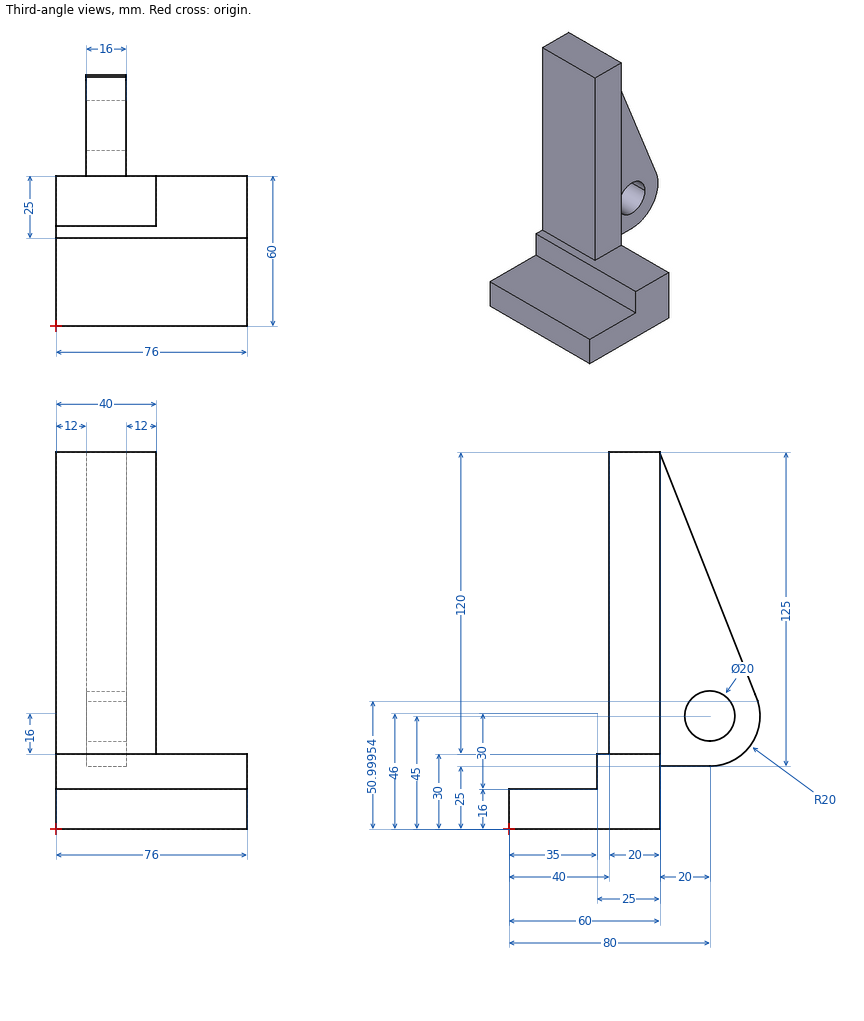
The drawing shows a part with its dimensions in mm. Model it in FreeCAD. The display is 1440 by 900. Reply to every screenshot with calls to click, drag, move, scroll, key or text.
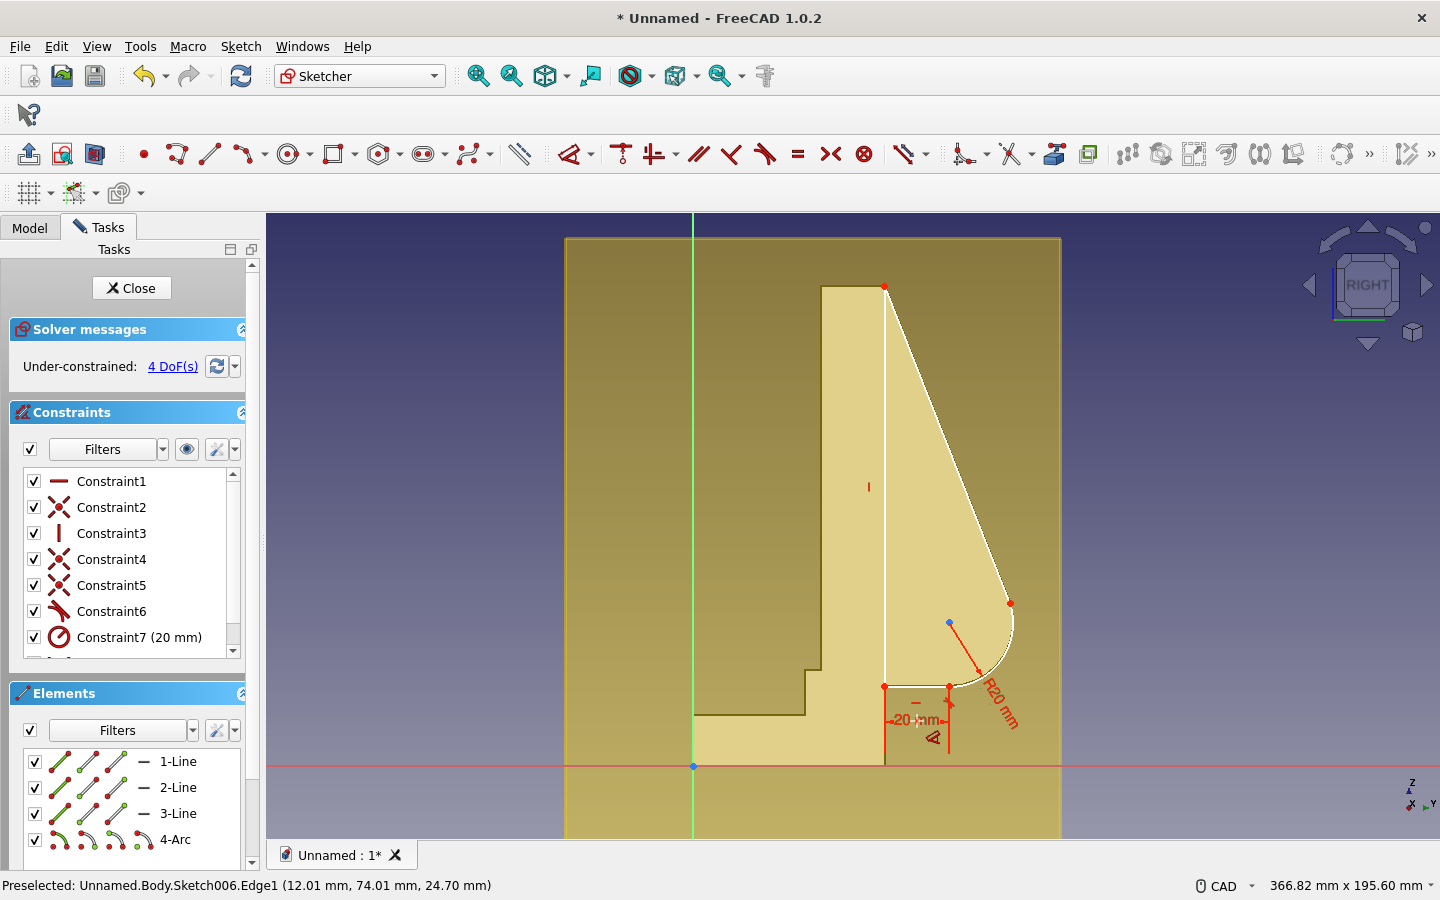
click(885, 567)
click(919, 487)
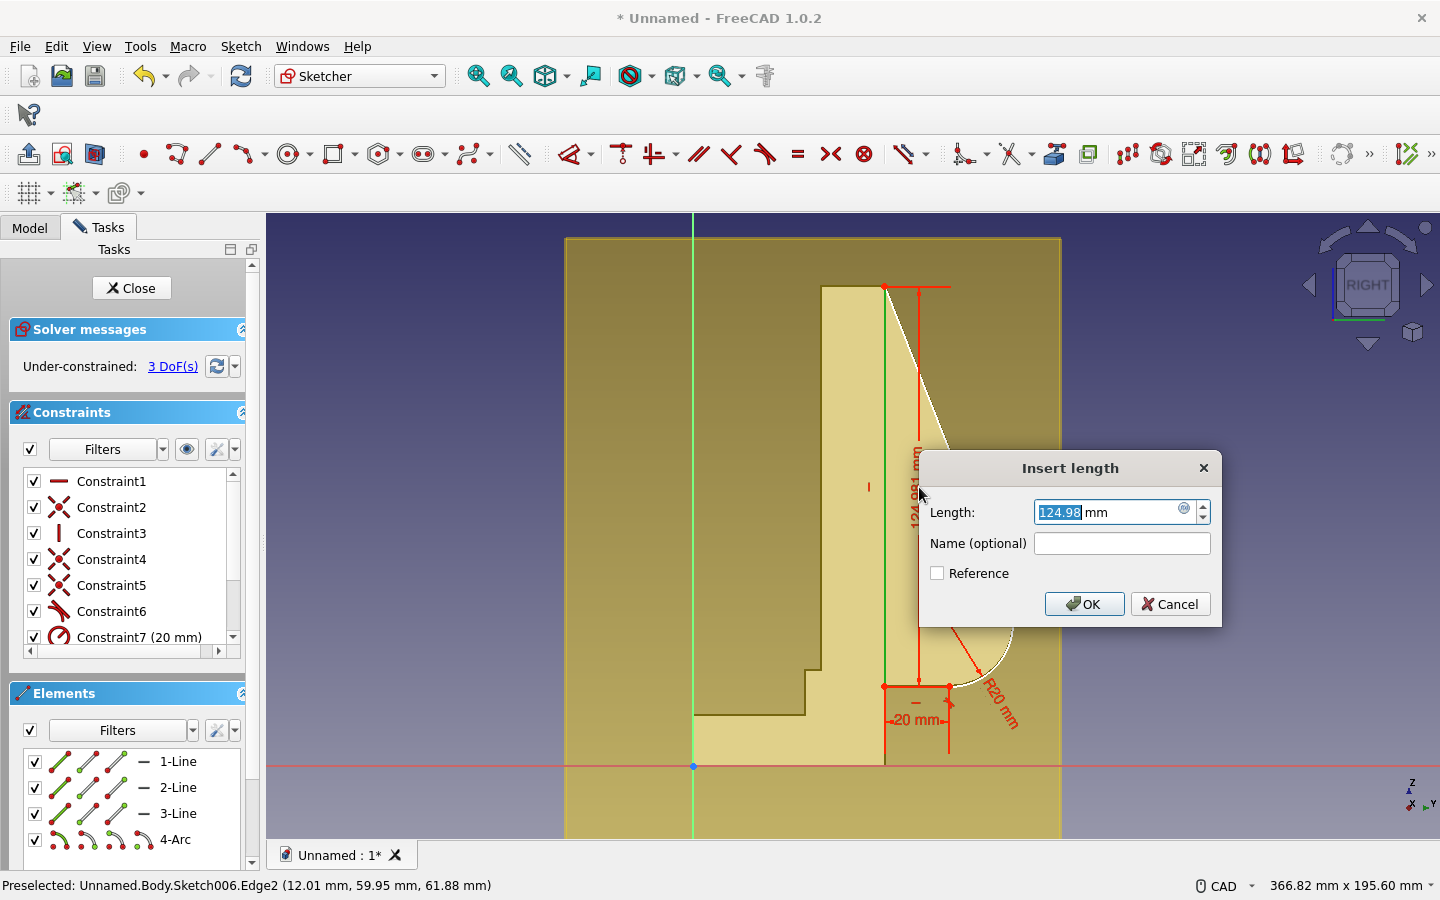
text(125)
key(Return)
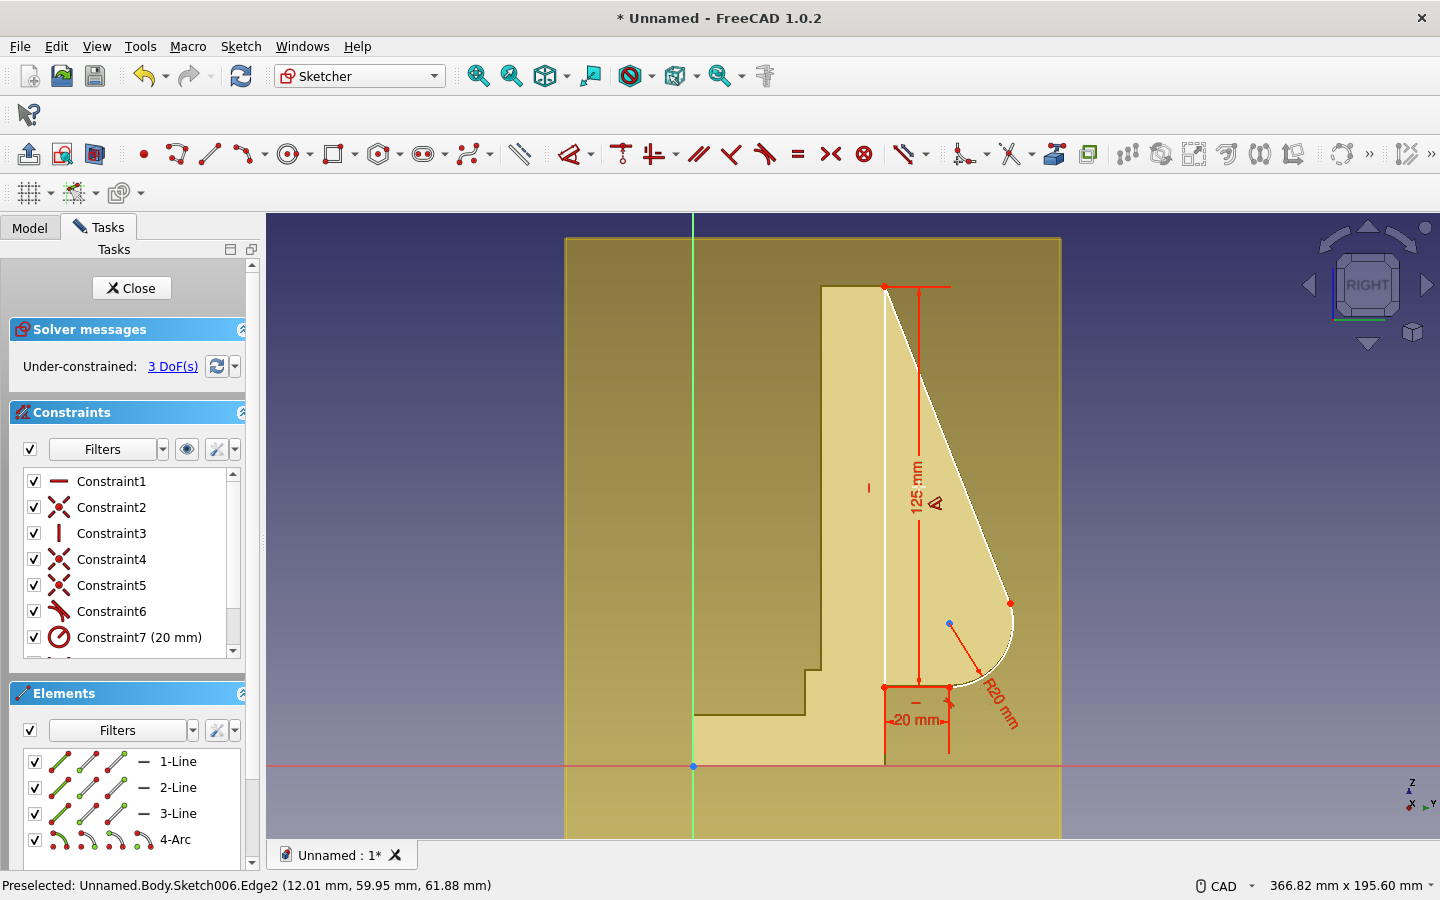
click(949, 687)
click(821, 800)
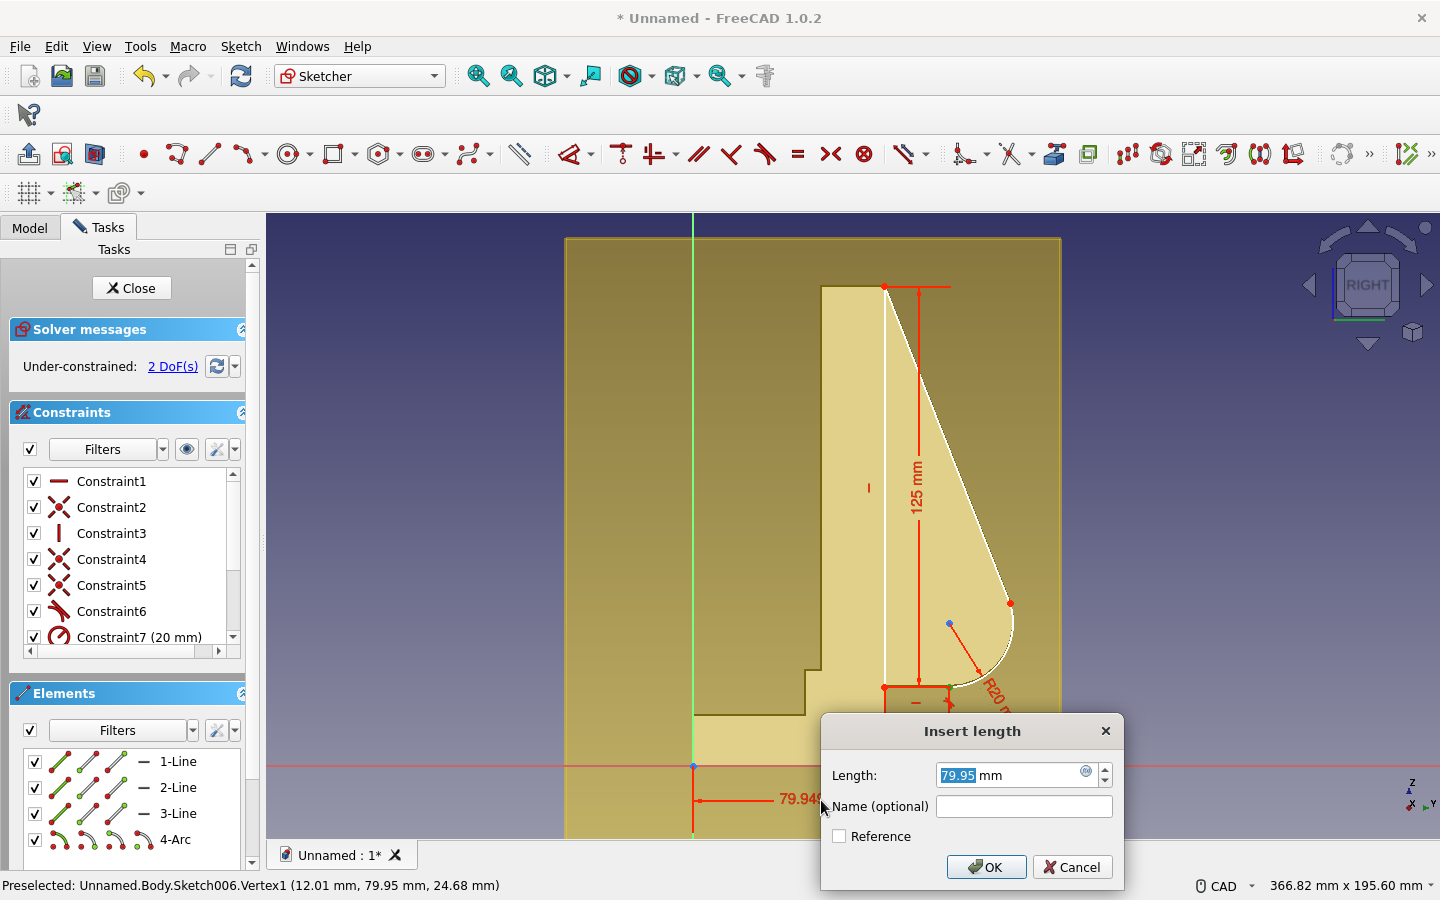
text(80)
key(Return)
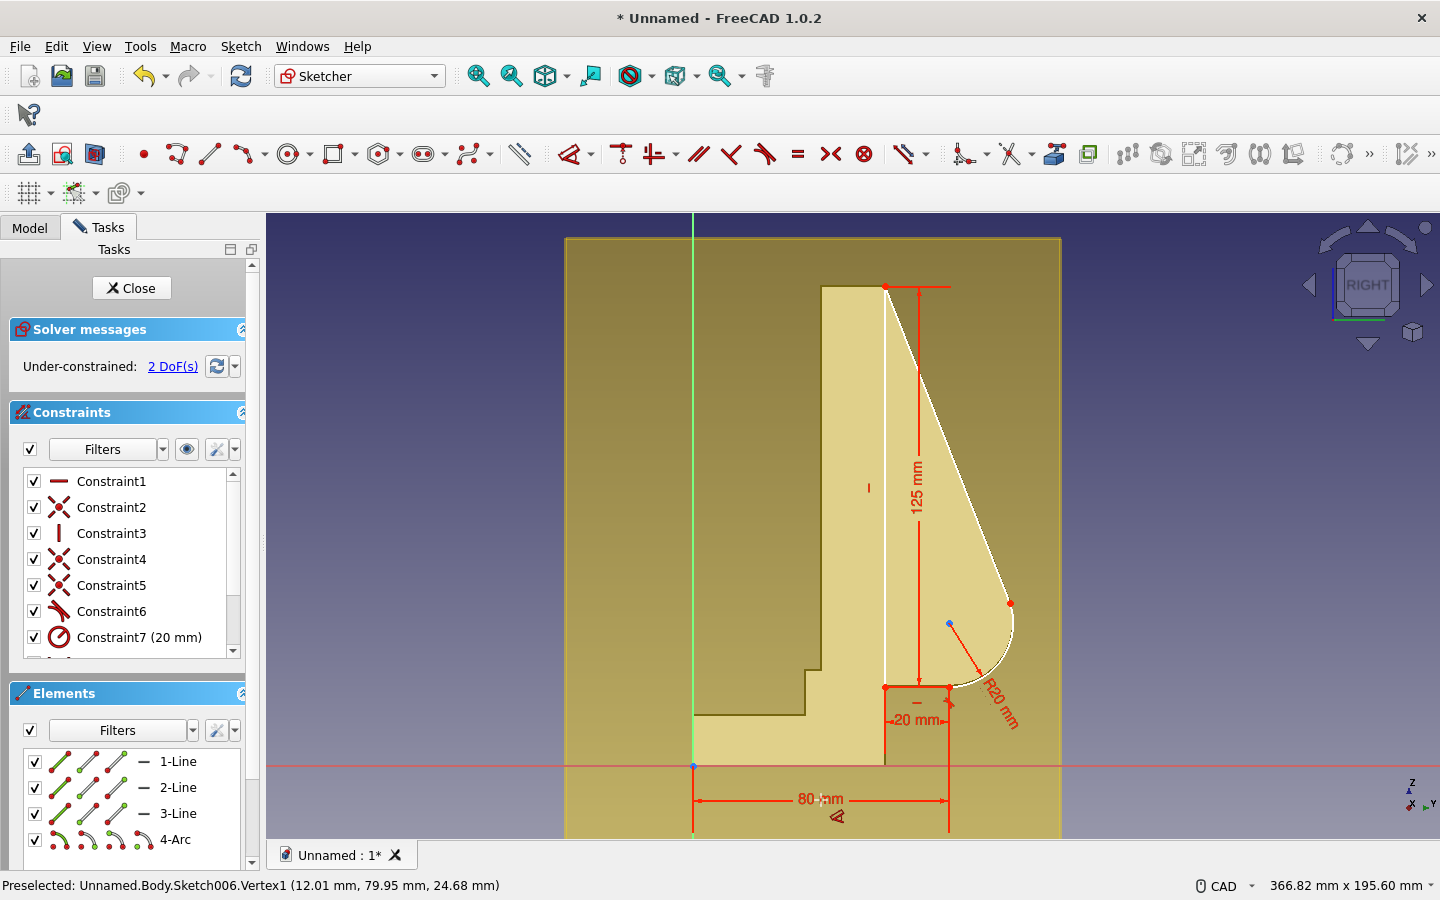
click(949, 687)
click(659, 727)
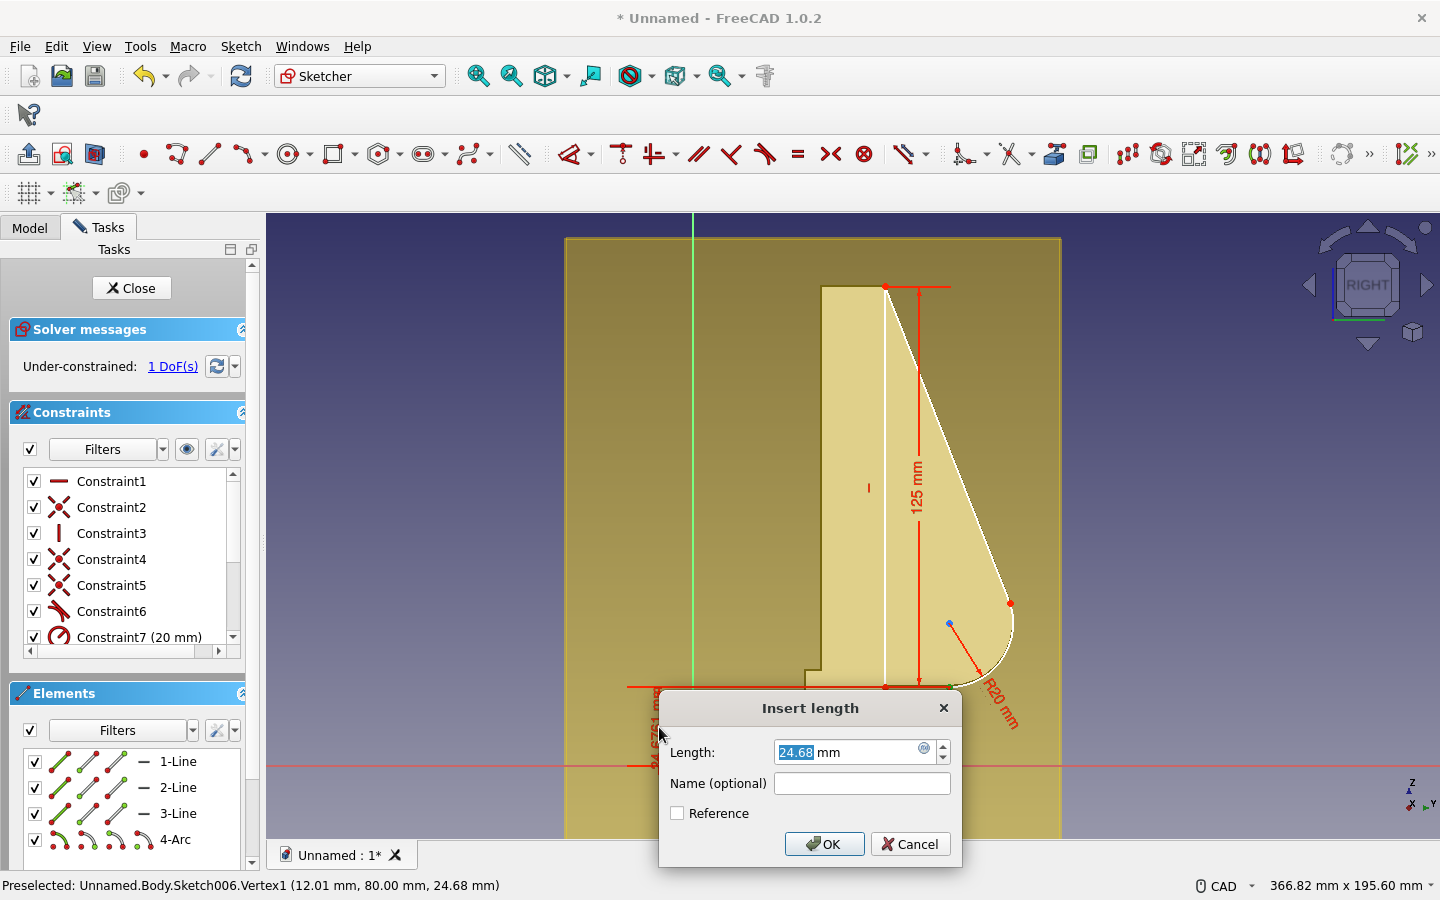
text(25)
key(Return)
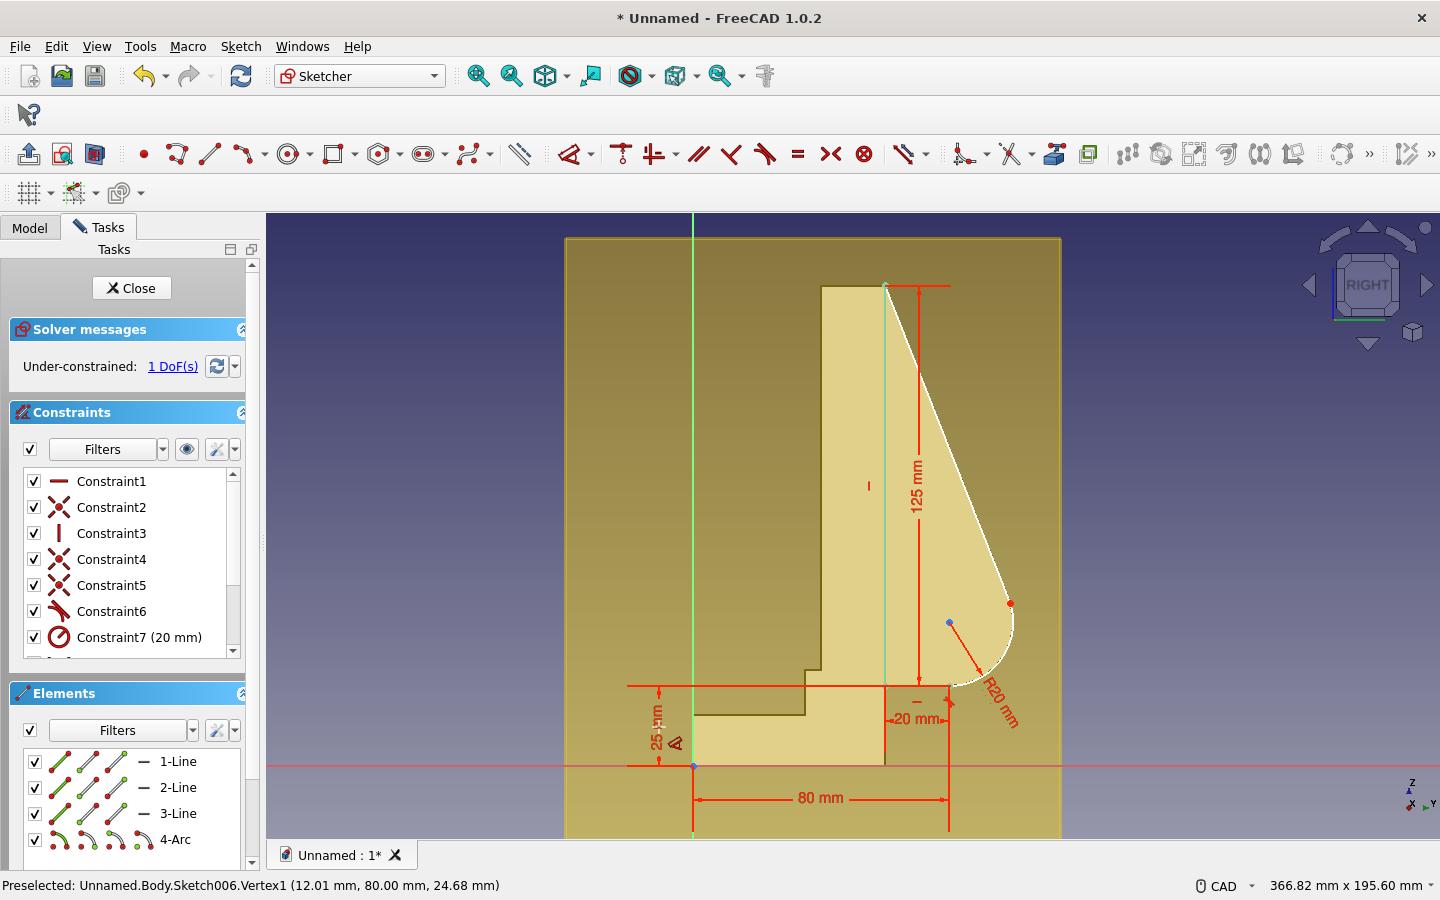
click(1011, 604)
click(1045, 648)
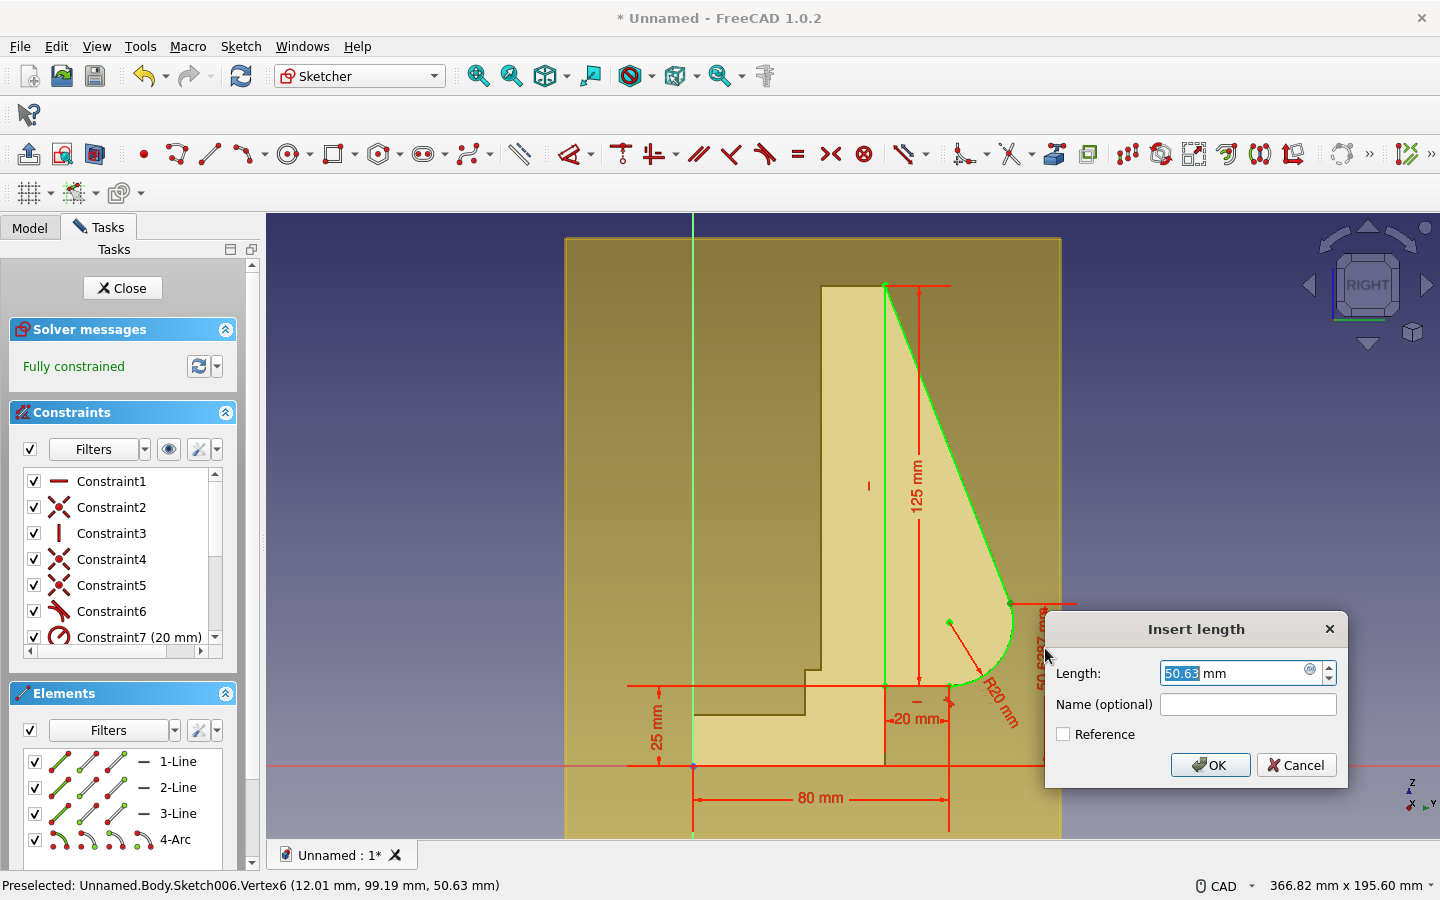
text(50.99954)
key(Return)
key(Escape)